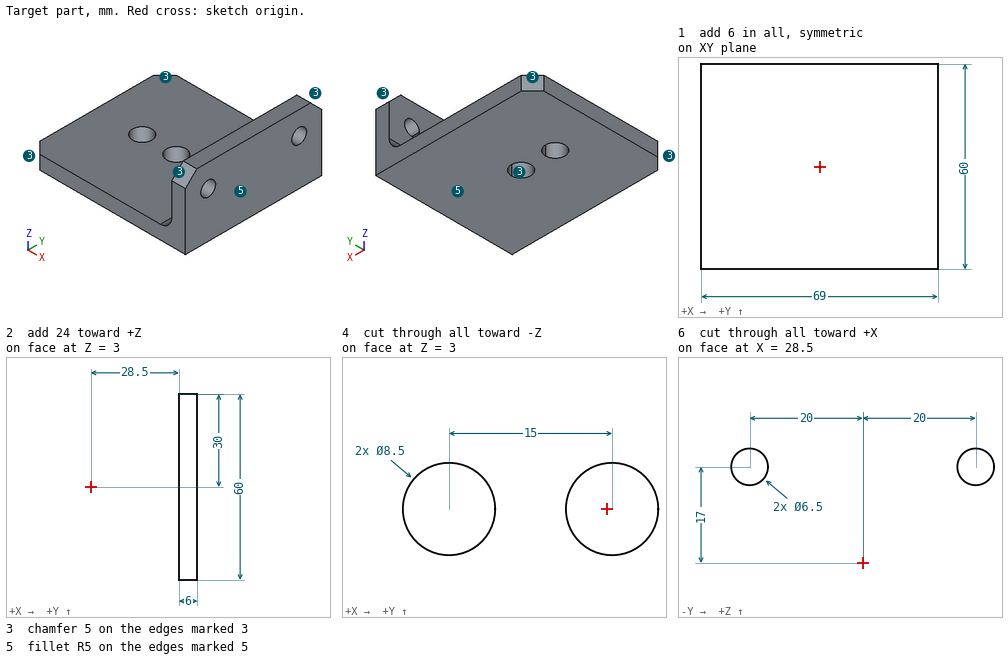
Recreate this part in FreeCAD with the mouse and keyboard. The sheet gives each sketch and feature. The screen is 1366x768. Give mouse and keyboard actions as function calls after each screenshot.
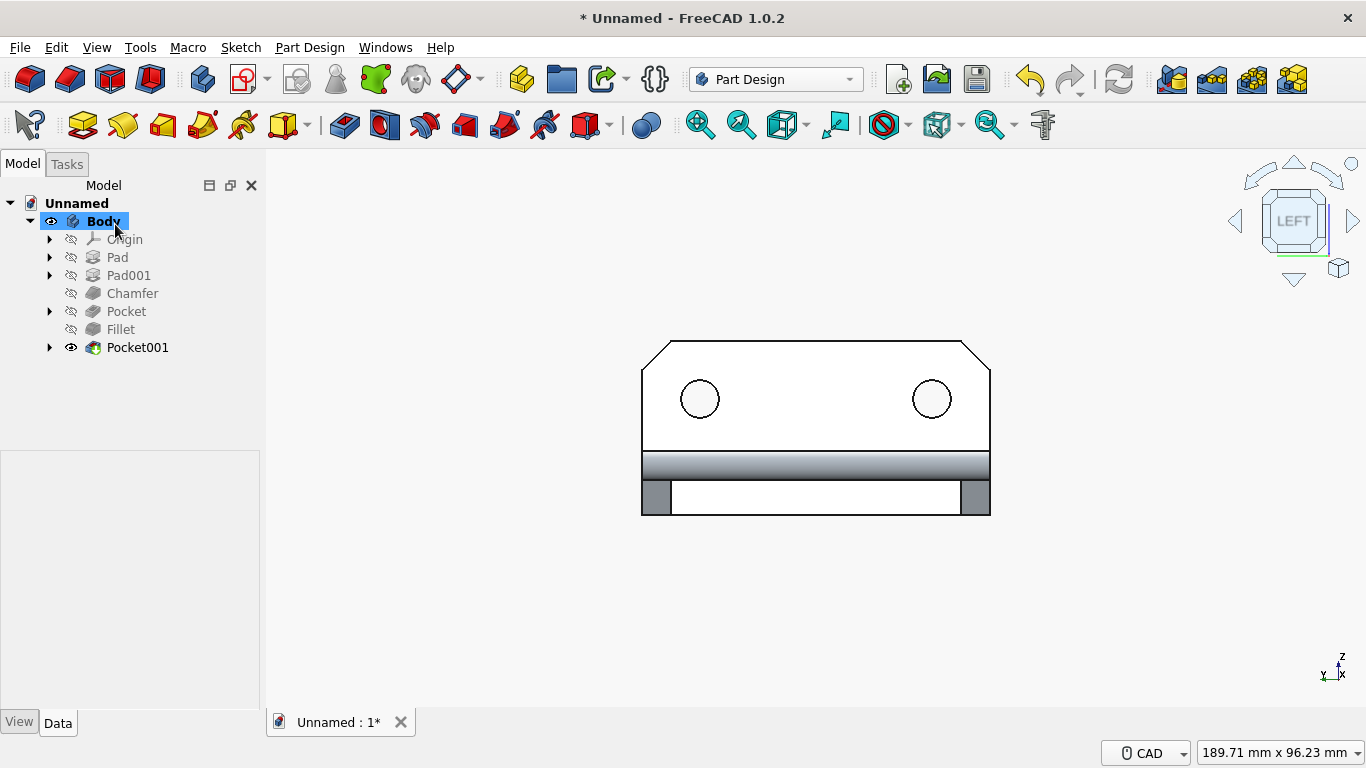
key(0)